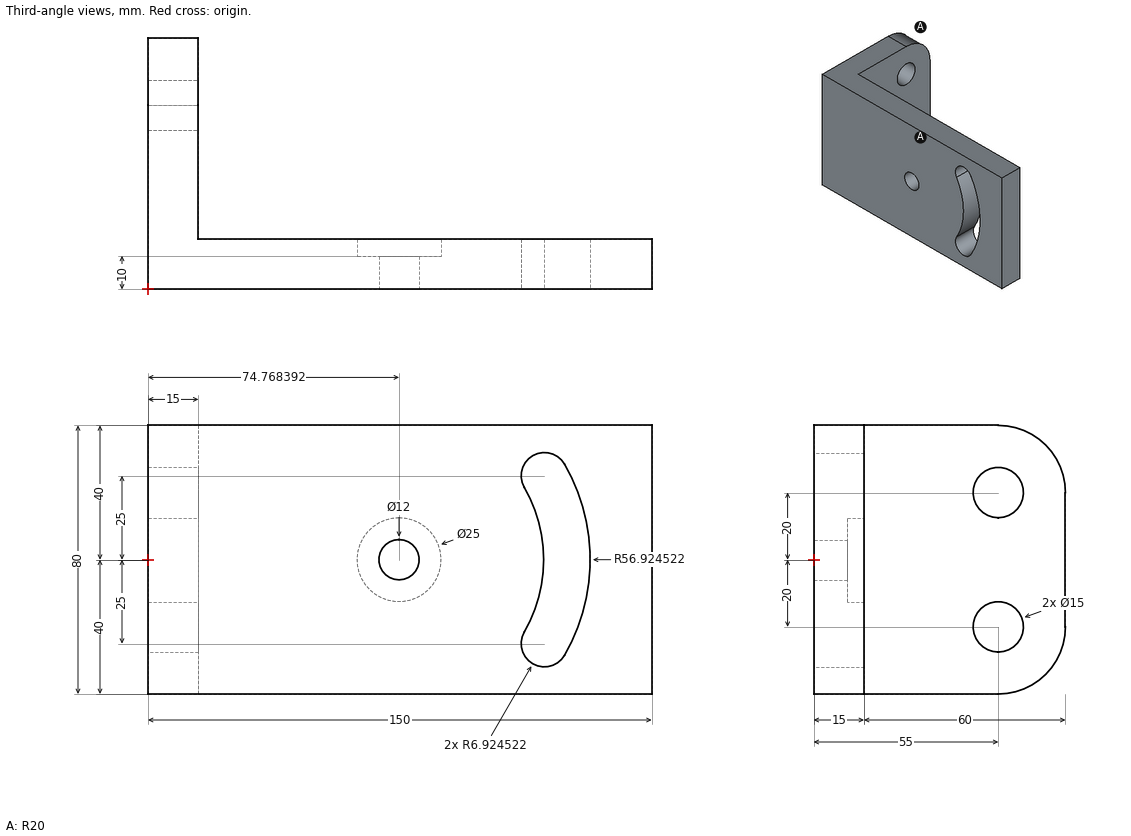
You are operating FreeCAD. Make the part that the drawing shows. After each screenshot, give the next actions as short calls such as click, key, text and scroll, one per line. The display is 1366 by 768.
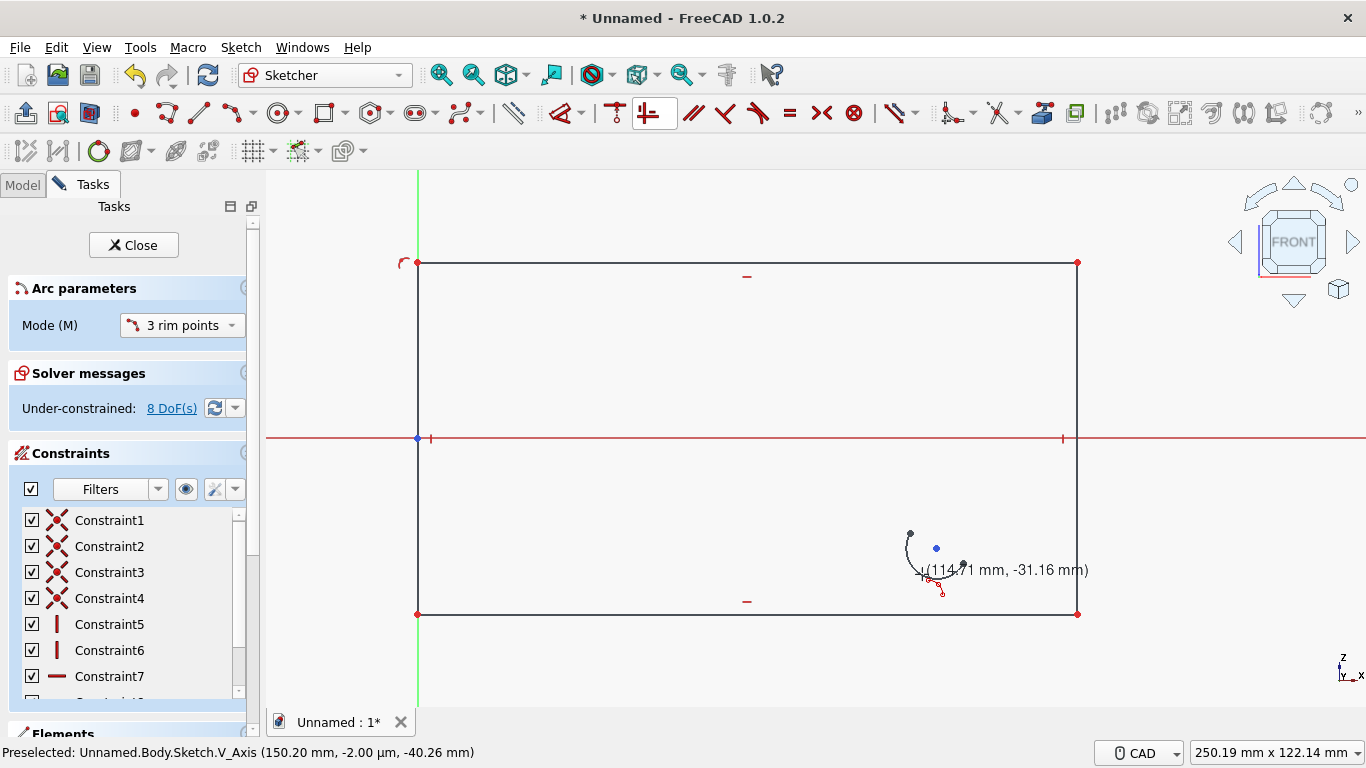
click(963, 564)
click(963, 313)
click(995, 464)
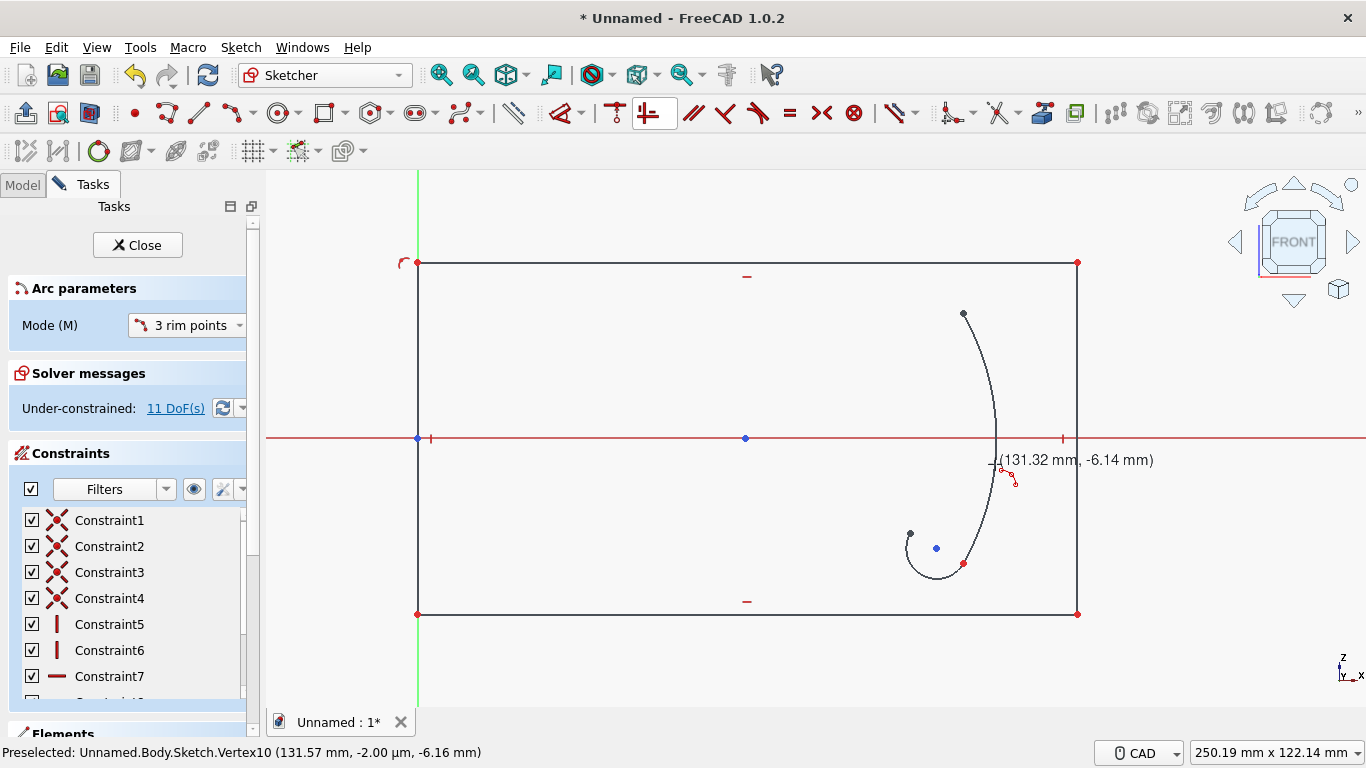
click(963, 314)
click(910, 343)
click(922, 302)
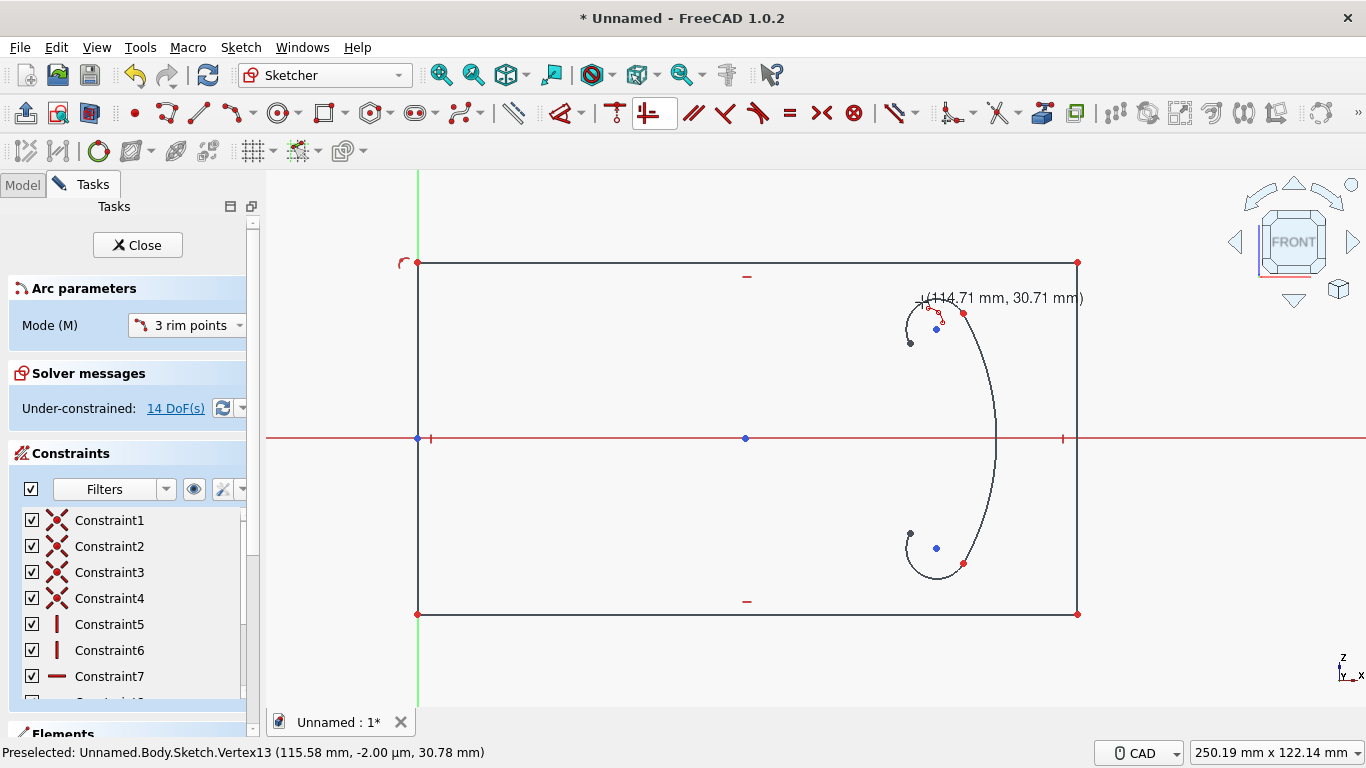
click(910, 344)
click(910, 534)
click(935, 458)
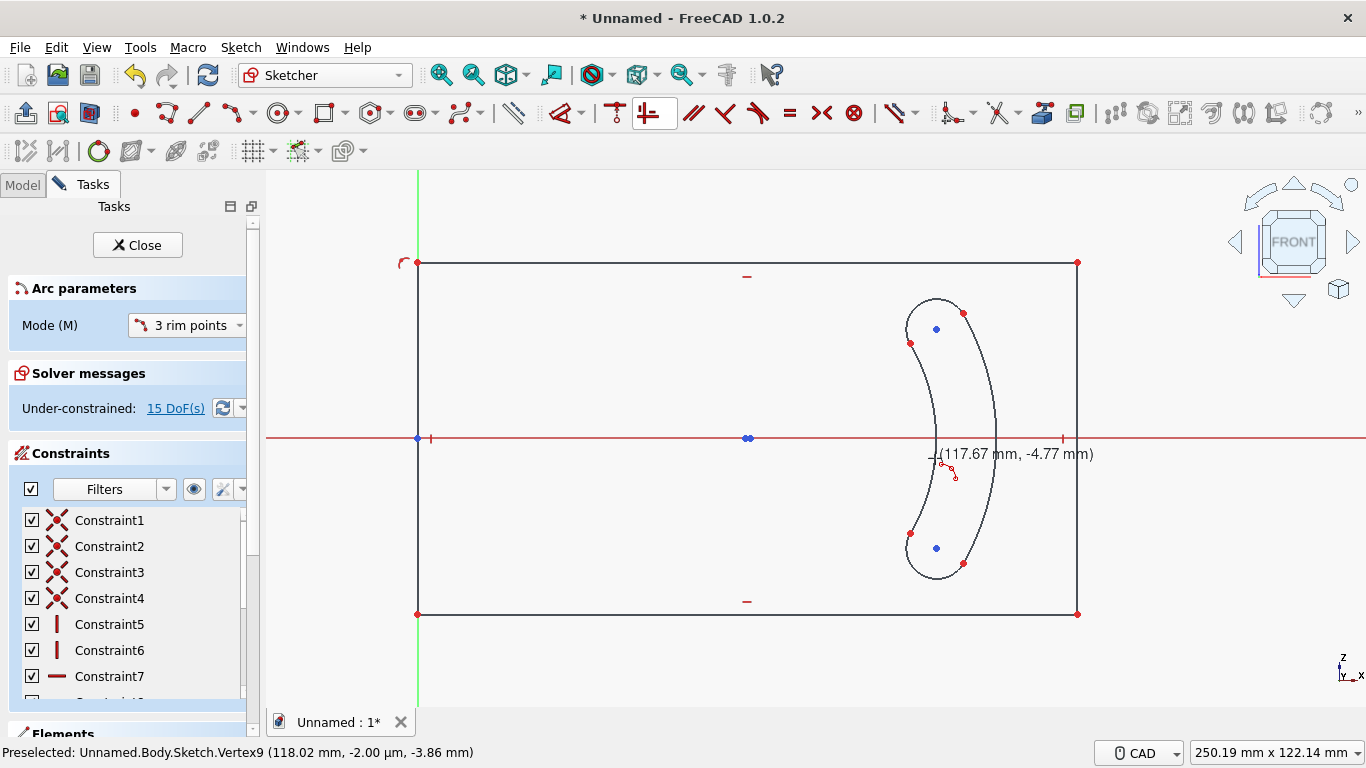
click(278, 114)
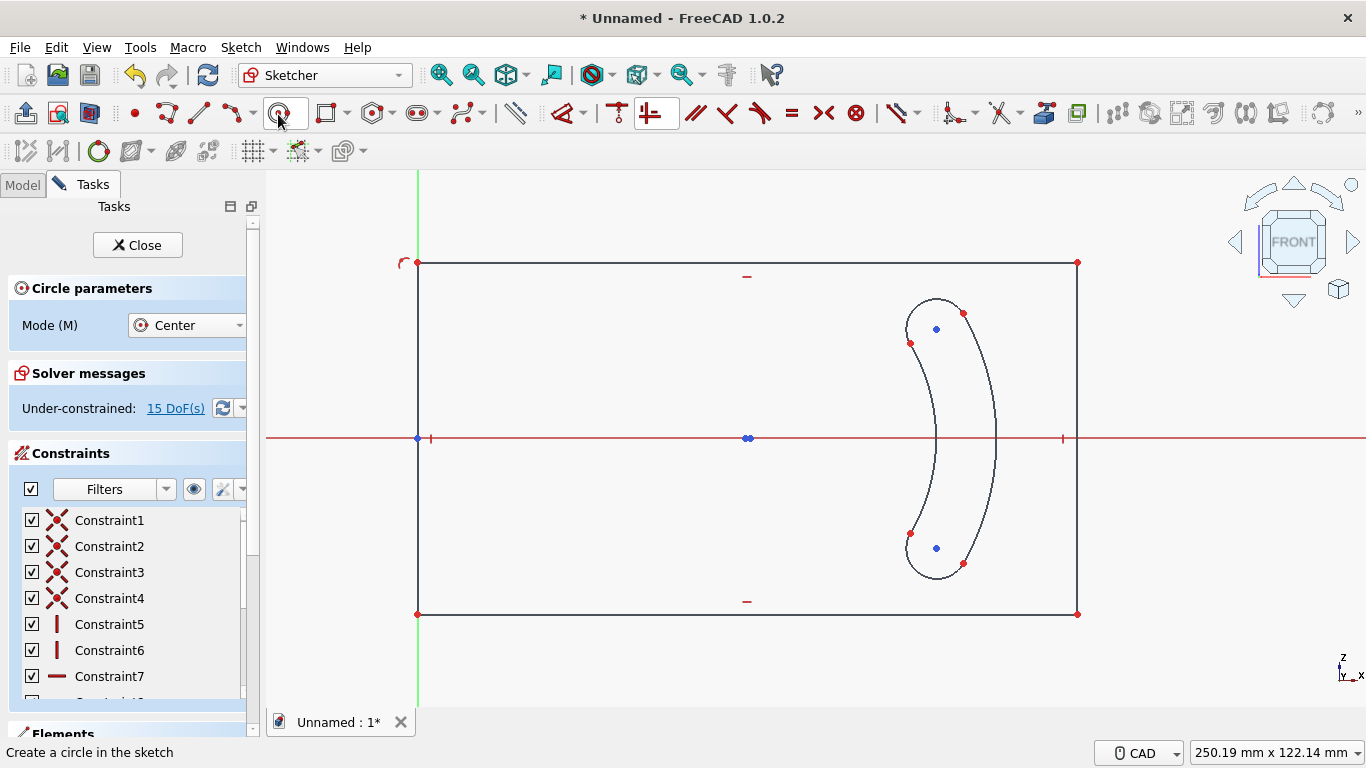
click(746, 438)
click(785, 399)
key(Escape)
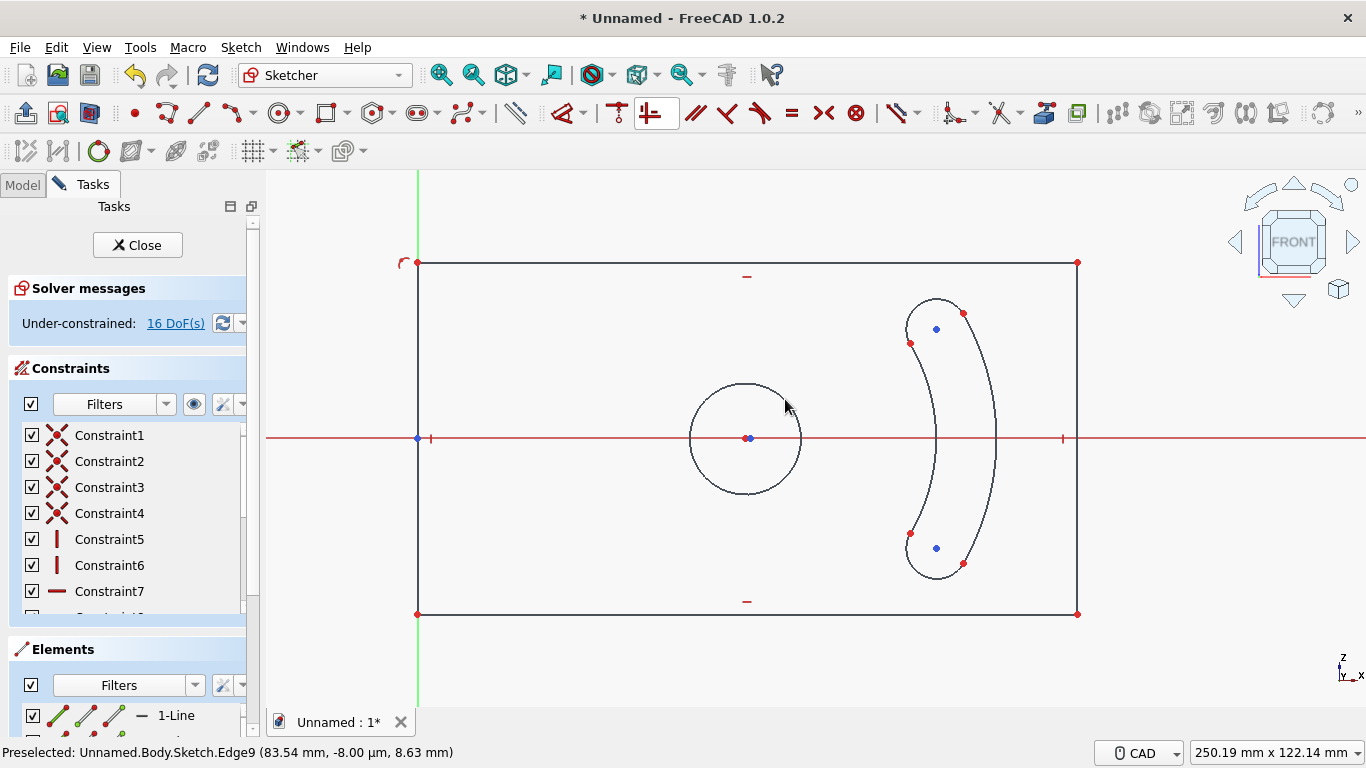
click(909, 561)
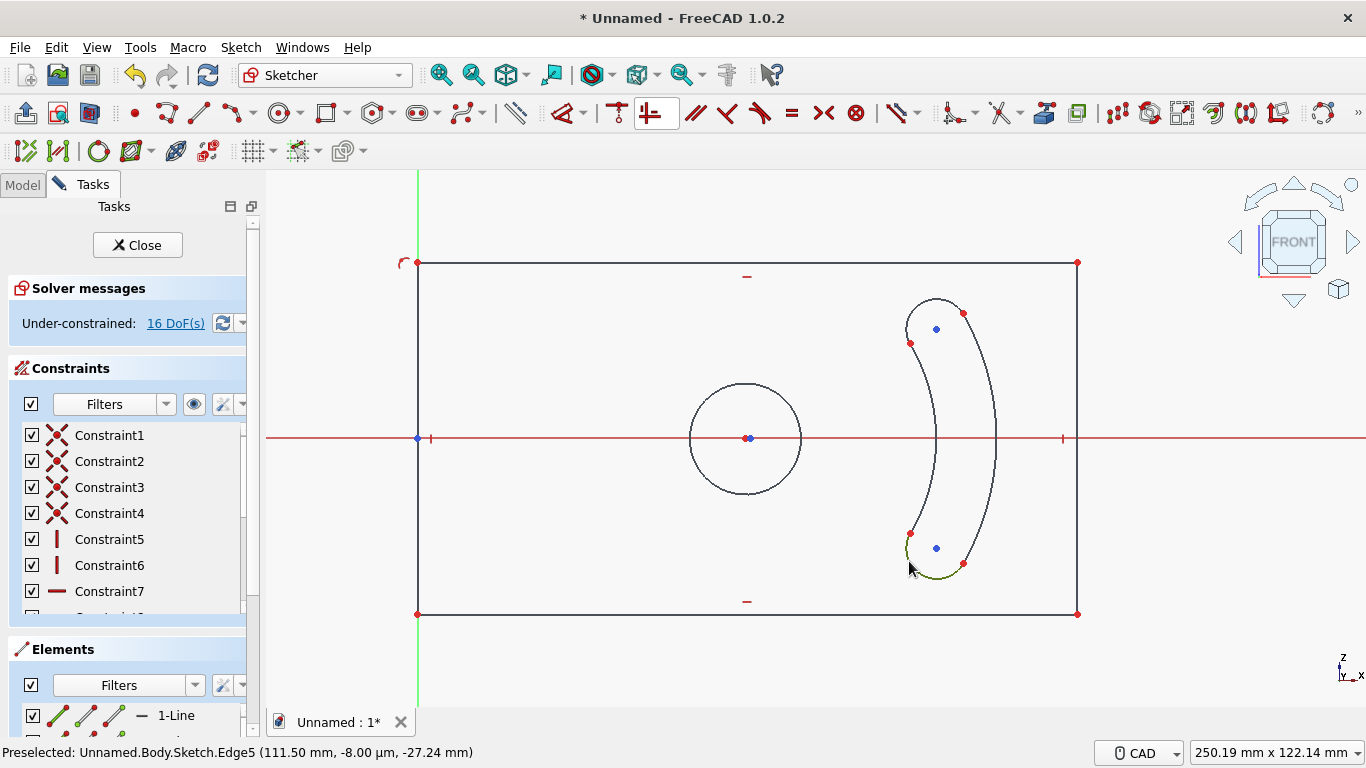
click(991, 491)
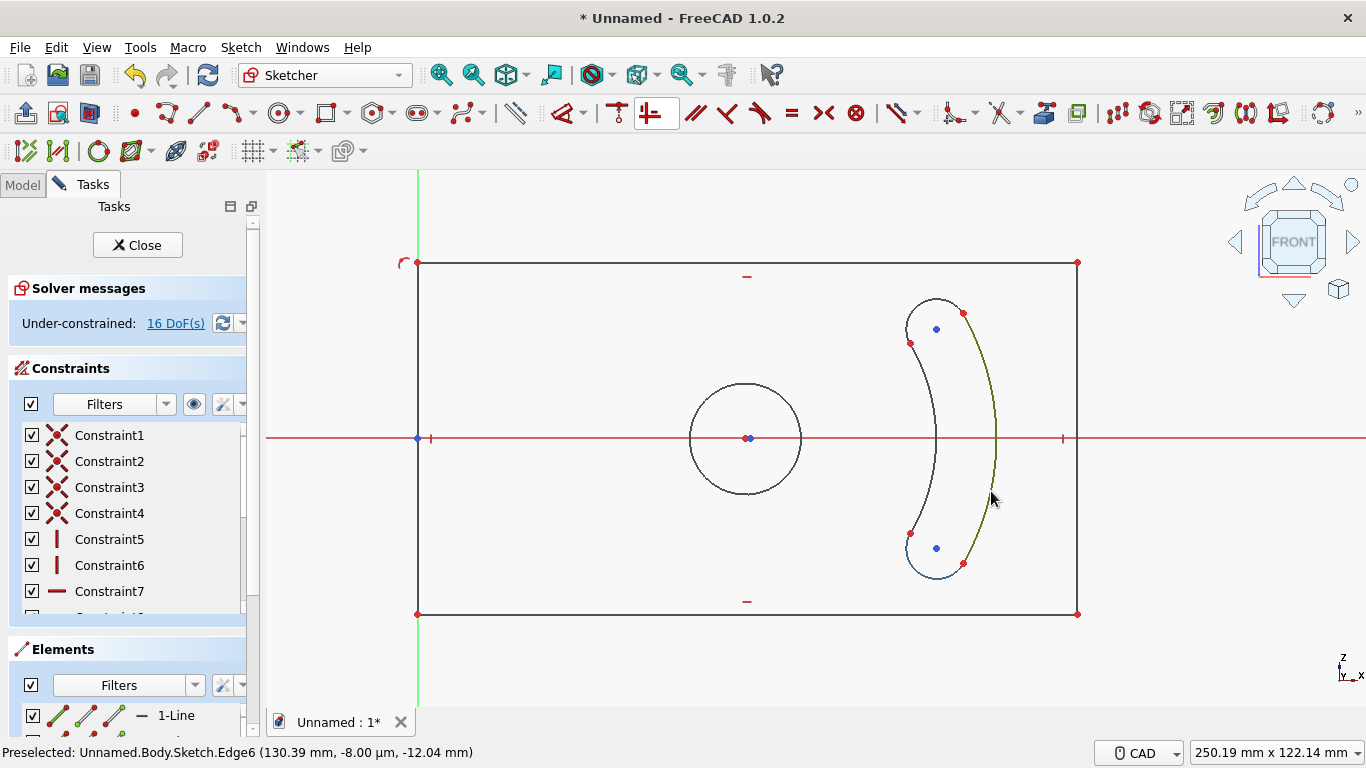
click(760, 114)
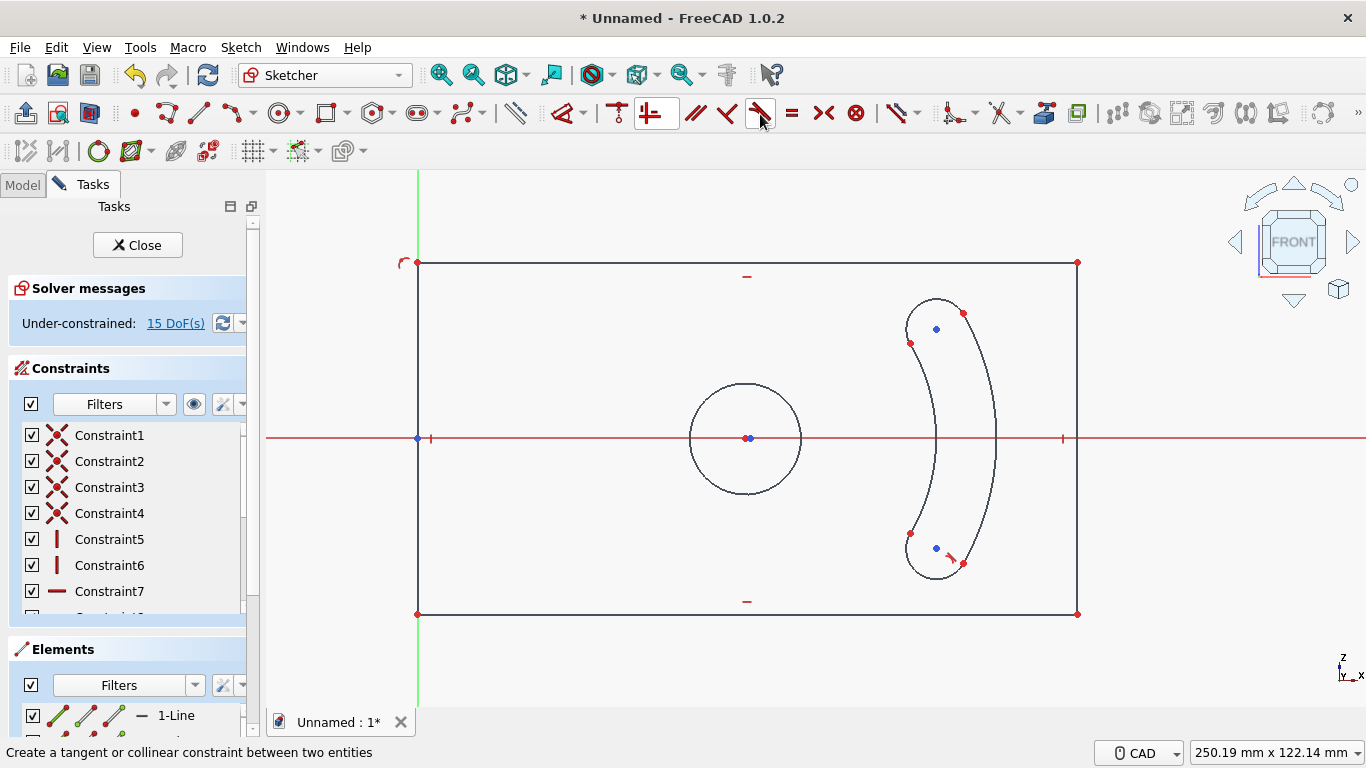
click(909, 562)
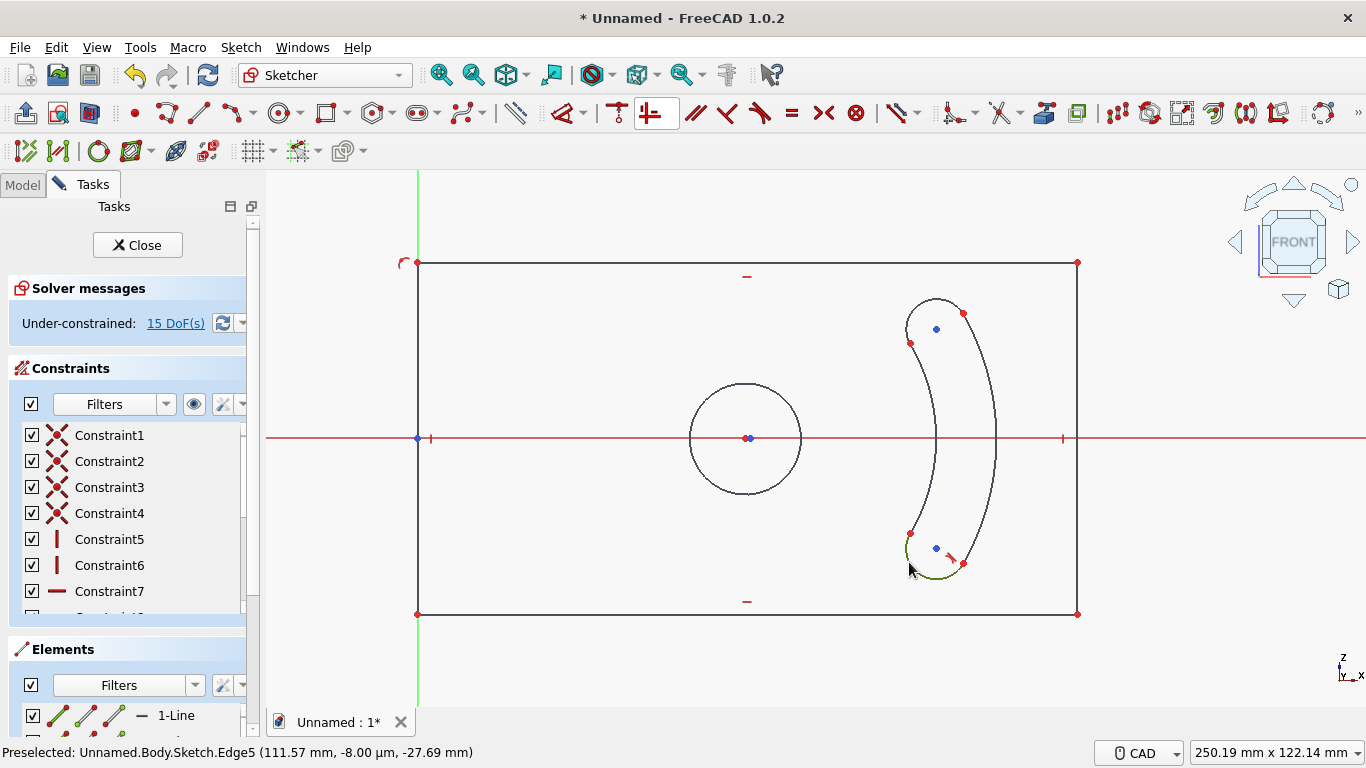
click(932, 479)